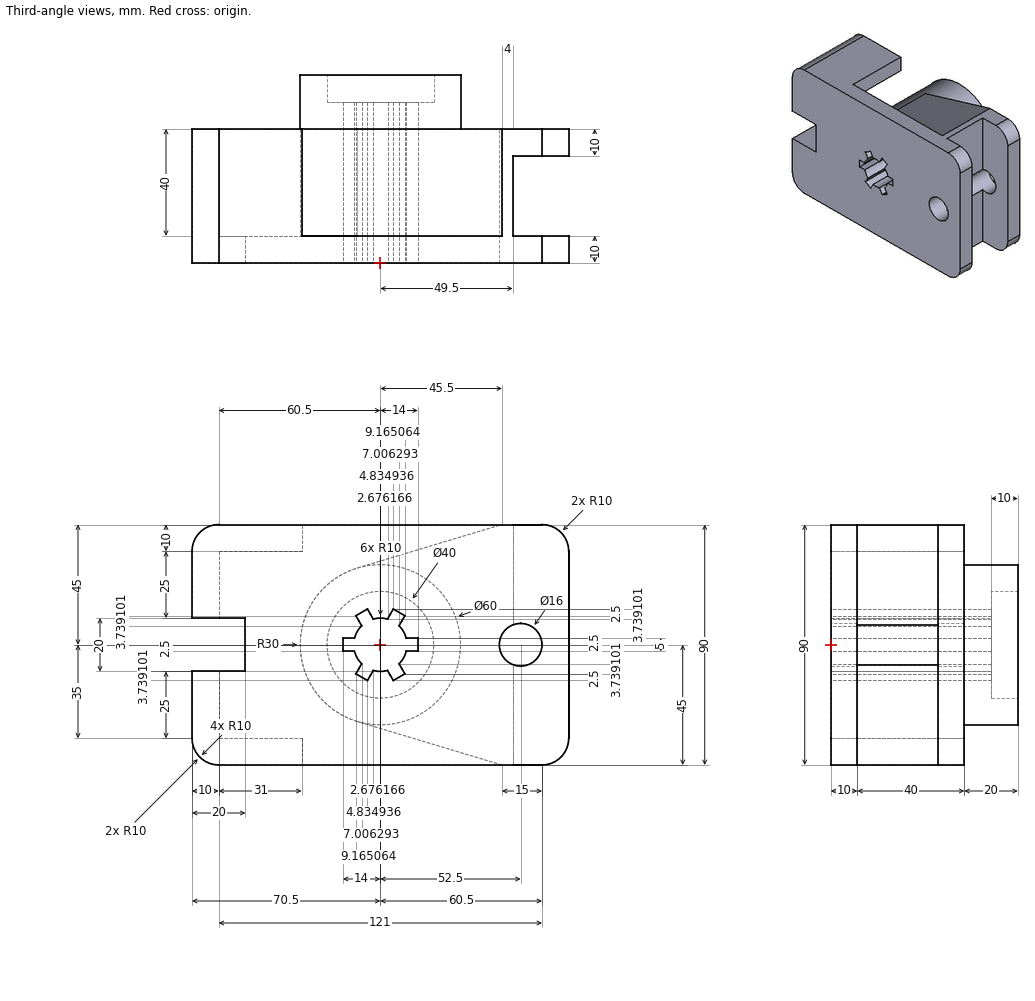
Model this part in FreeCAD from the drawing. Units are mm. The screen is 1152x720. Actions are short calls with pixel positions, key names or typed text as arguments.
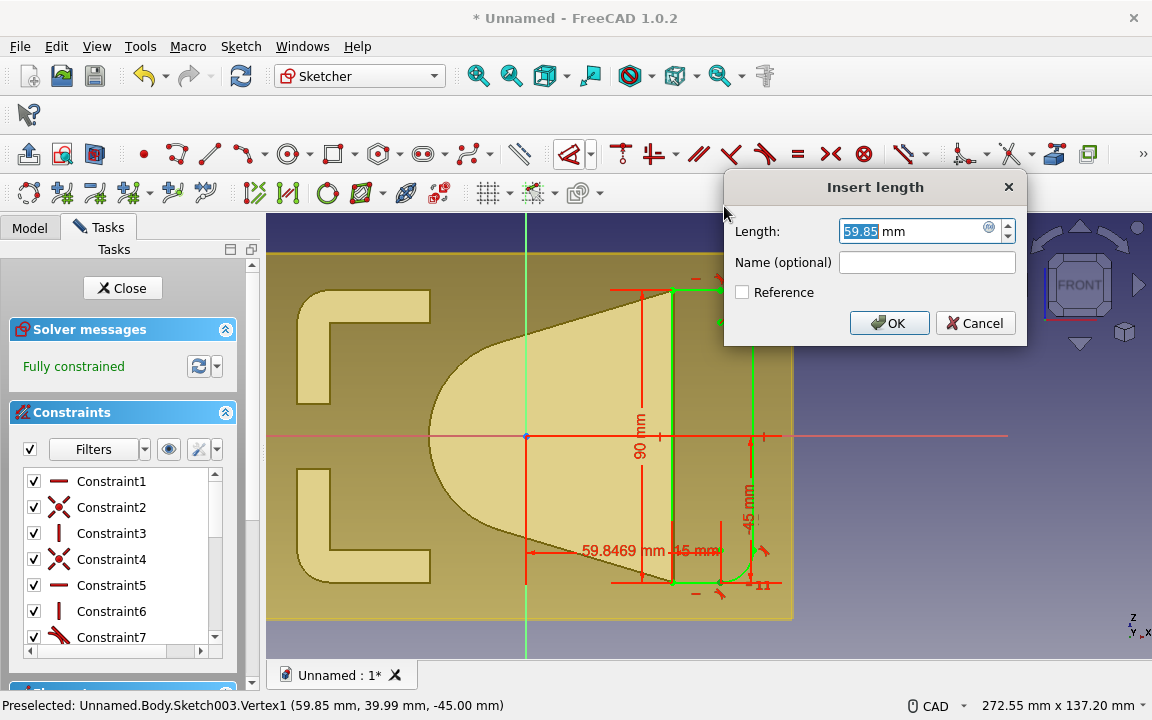
text(60.5)
key(Return)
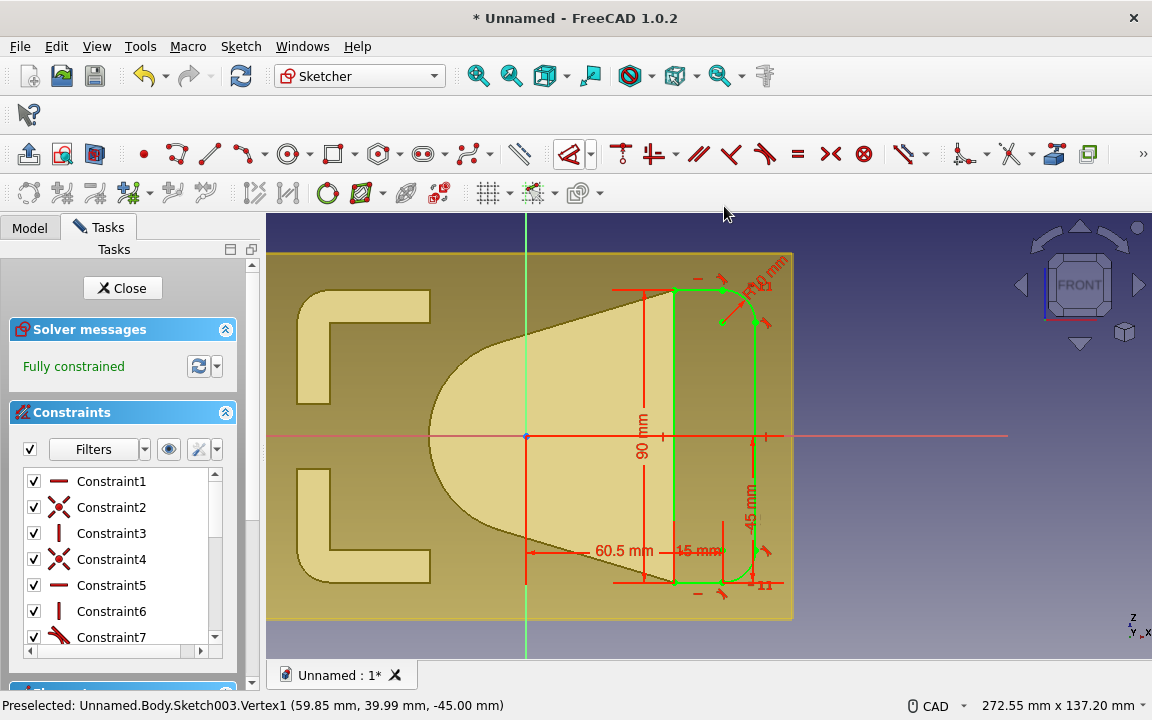
click(123, 288)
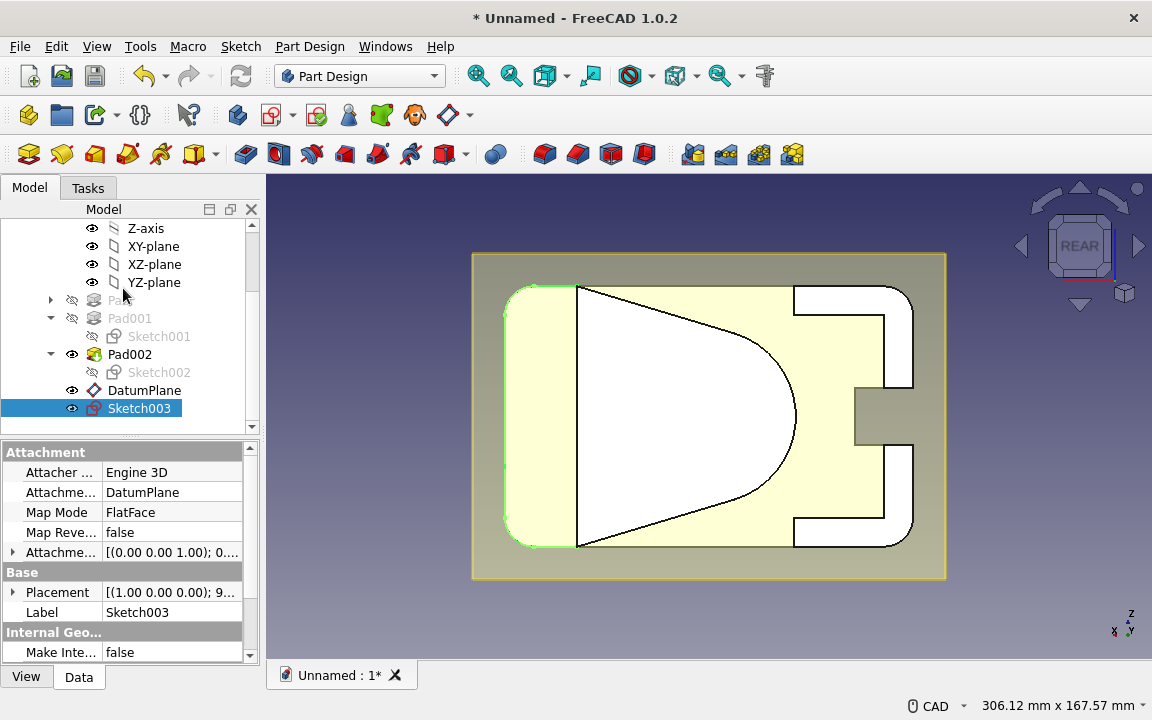
click(29, 154)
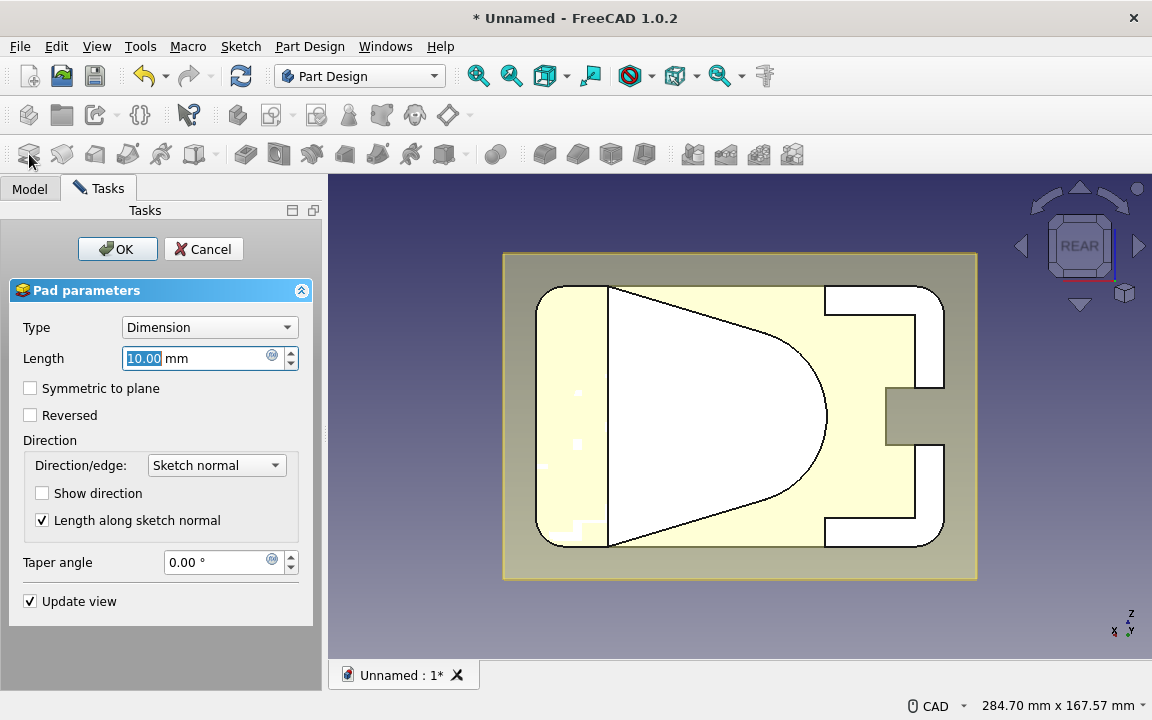
text(10)
key(Tab)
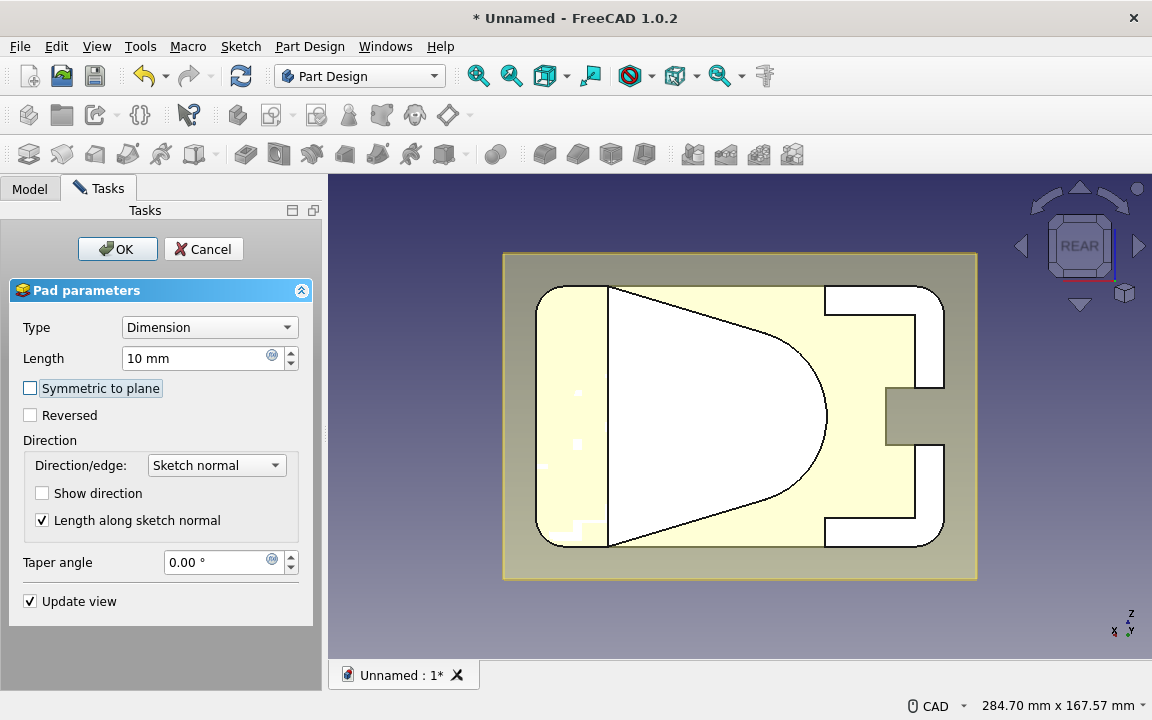
click(31, 415)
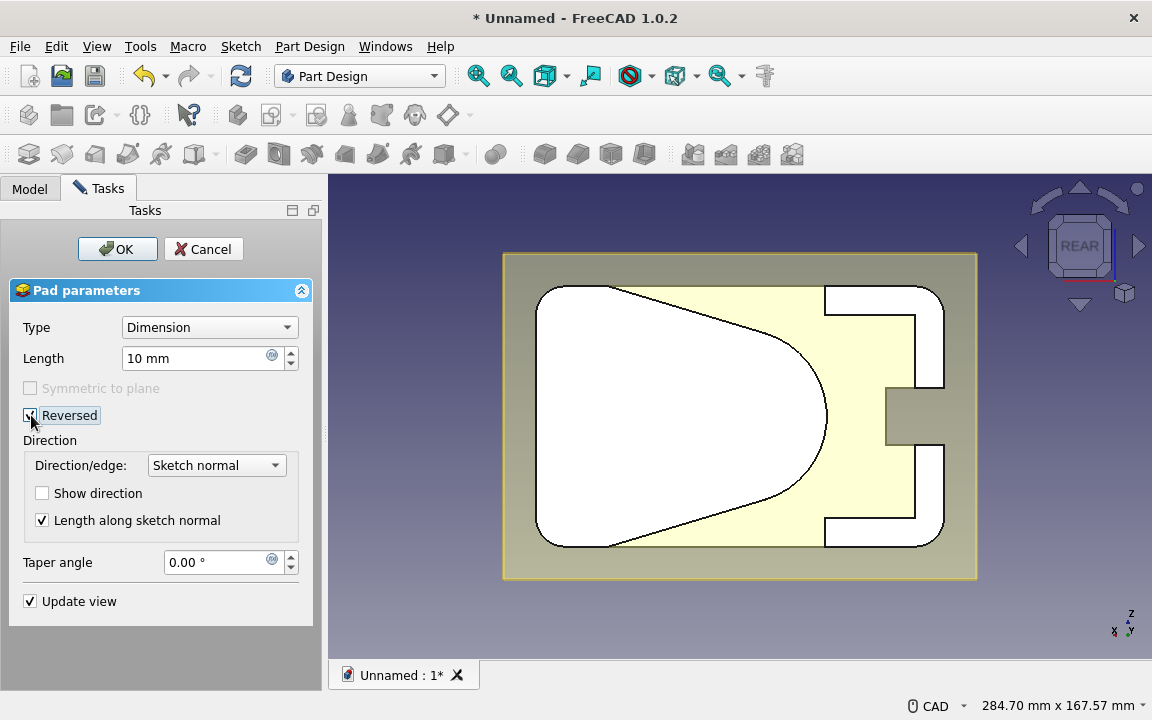
click(118, 249)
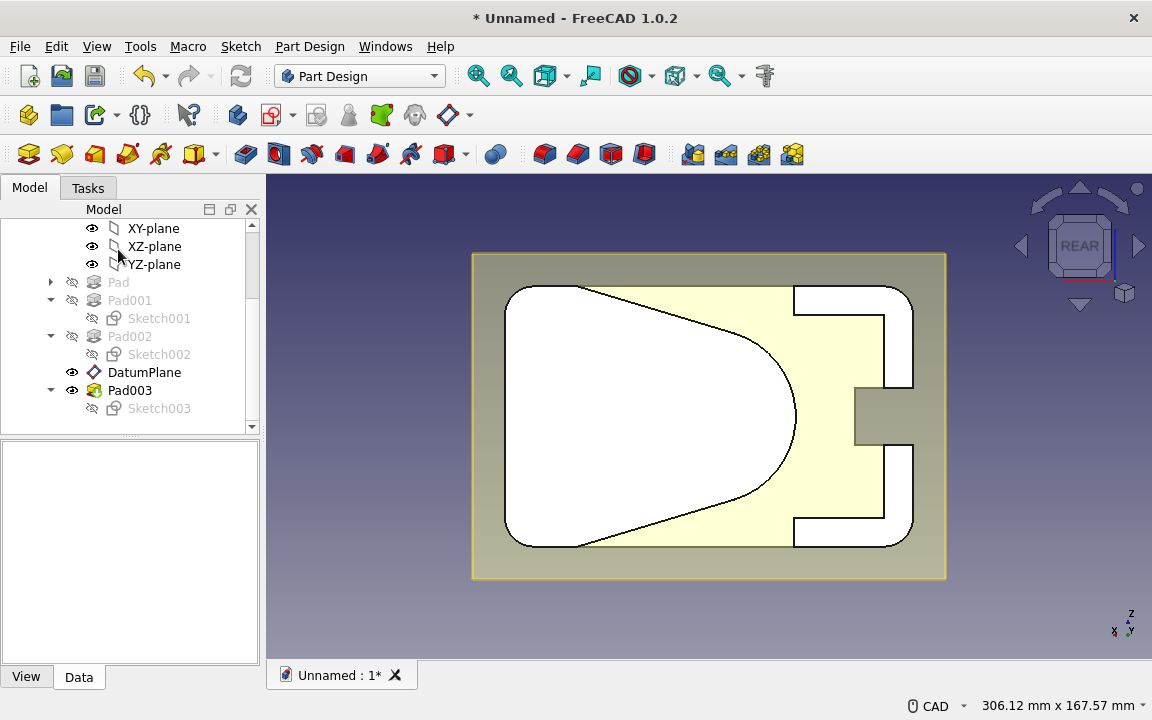
click(117, 372)
key(space)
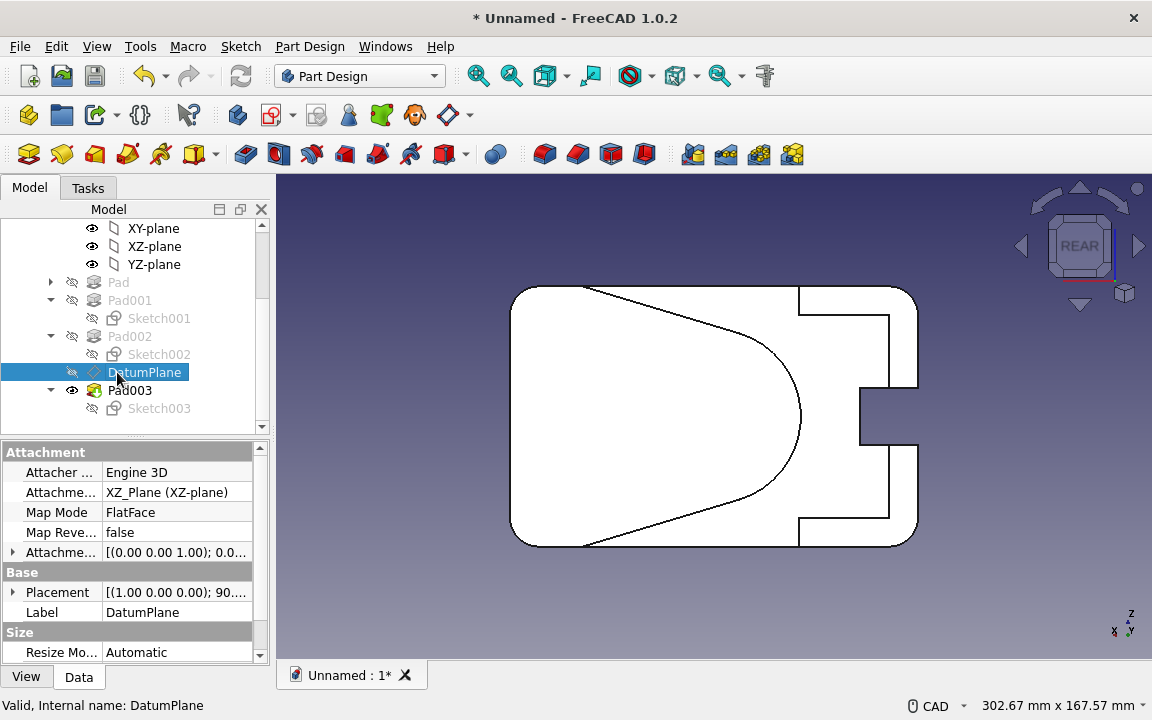
key(0)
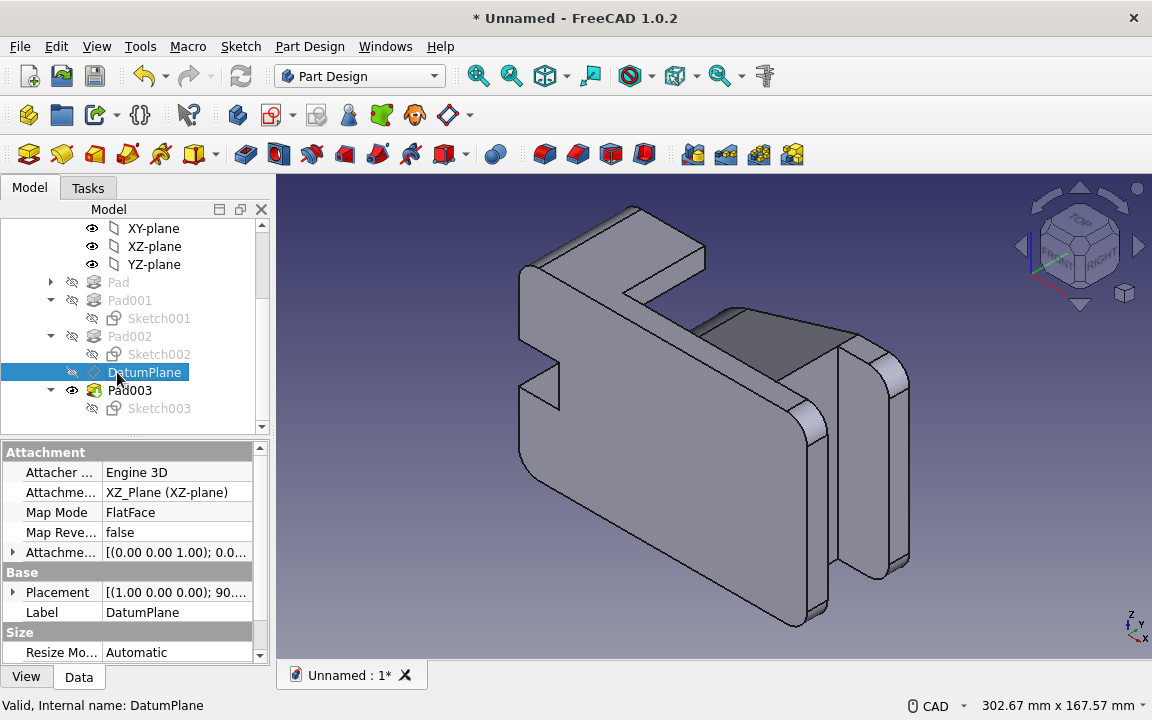
click(637, 231)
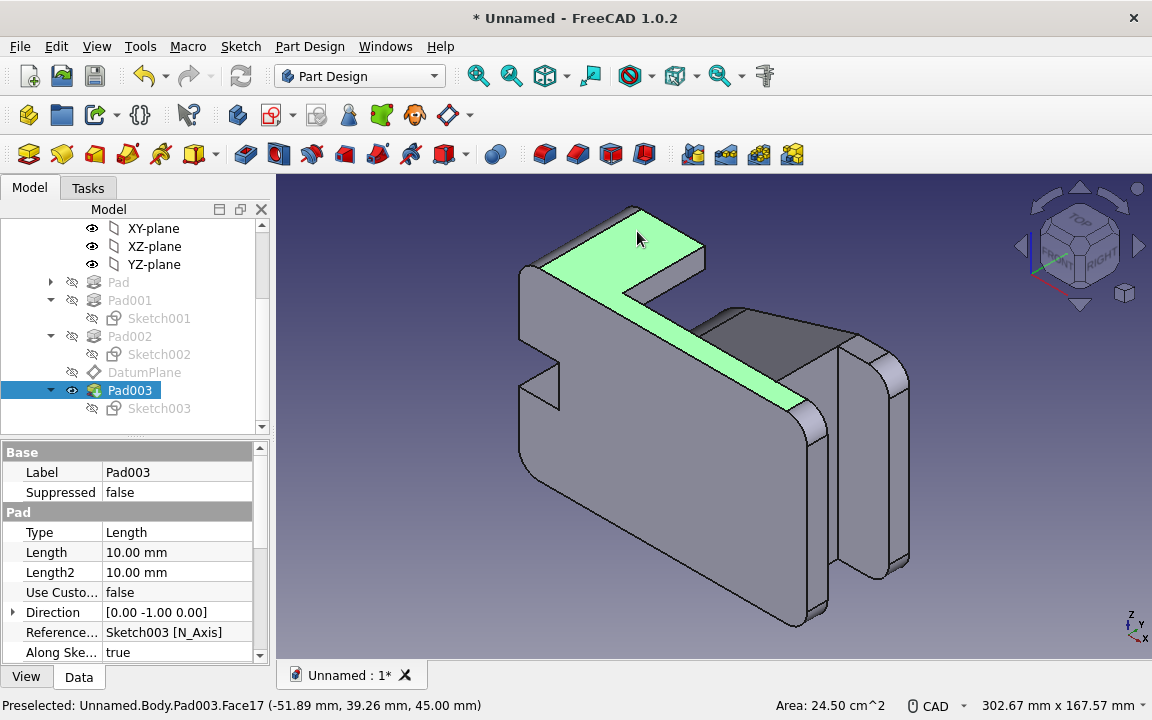
click(270, 116)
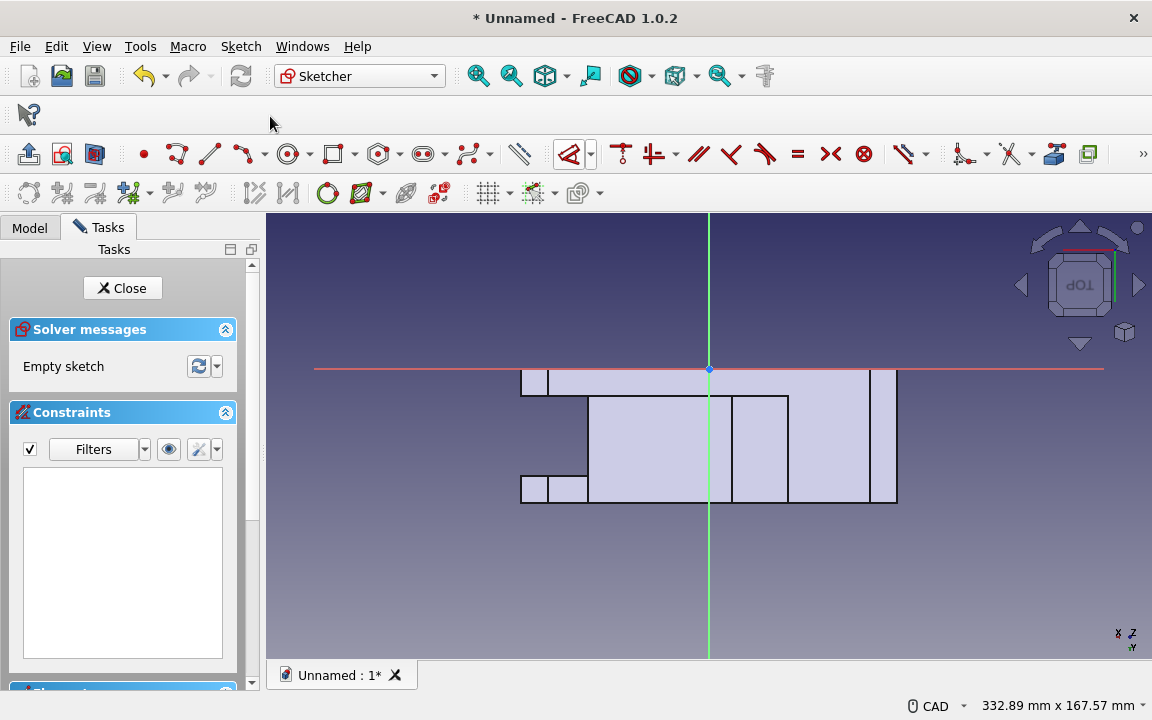
scroll(645, 436, up, 4)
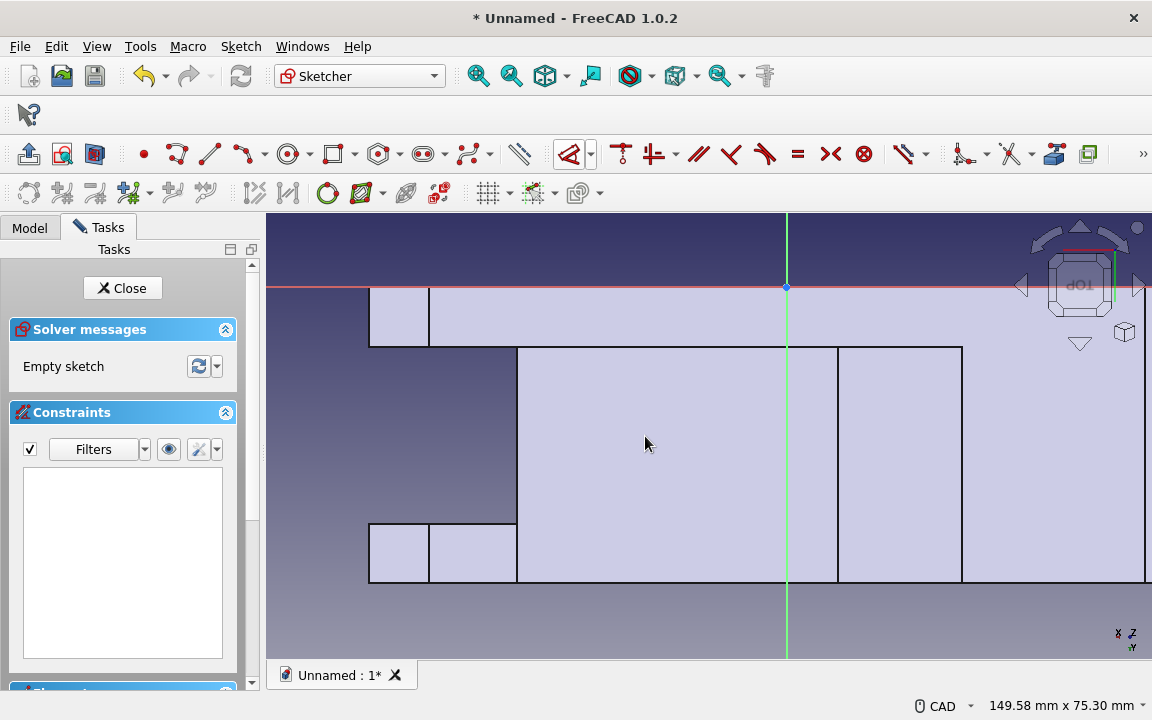
click(332, 154)